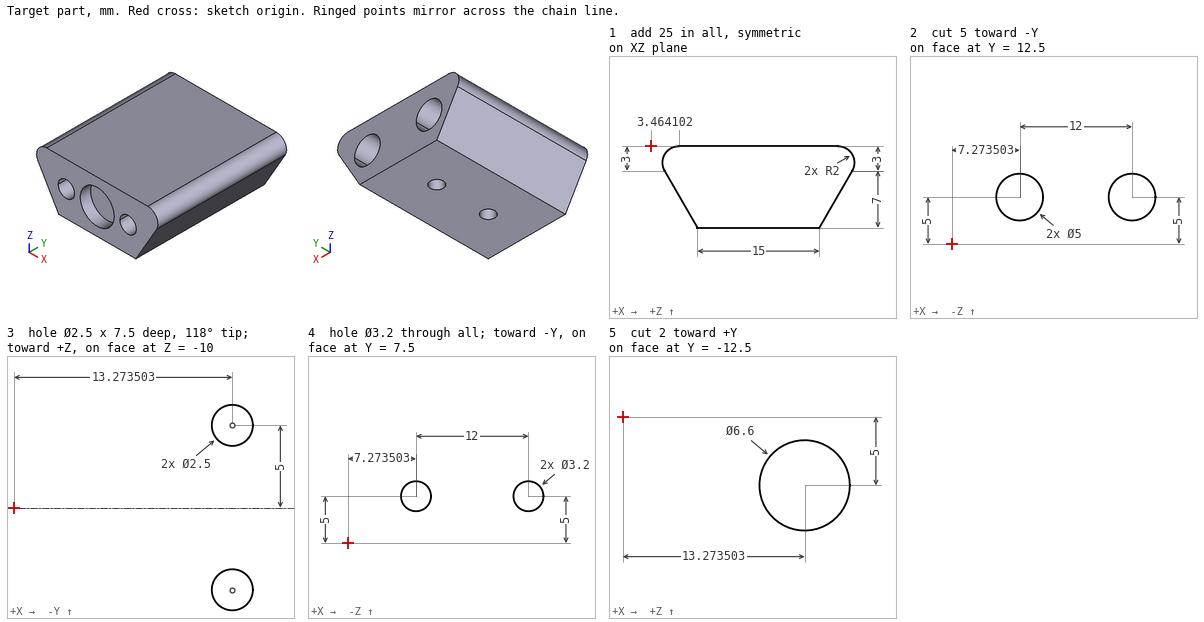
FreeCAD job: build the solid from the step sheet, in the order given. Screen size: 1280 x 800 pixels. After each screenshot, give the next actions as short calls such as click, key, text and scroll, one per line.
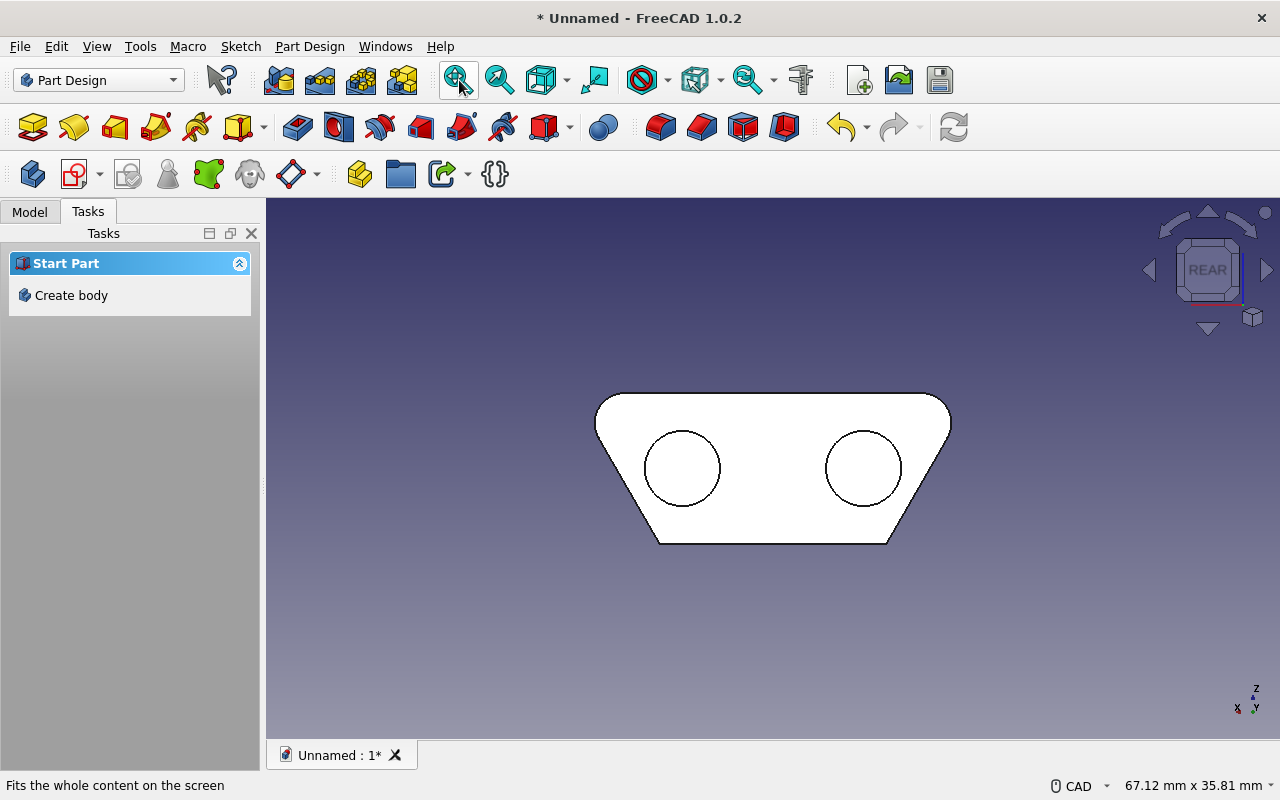
click(682, 467)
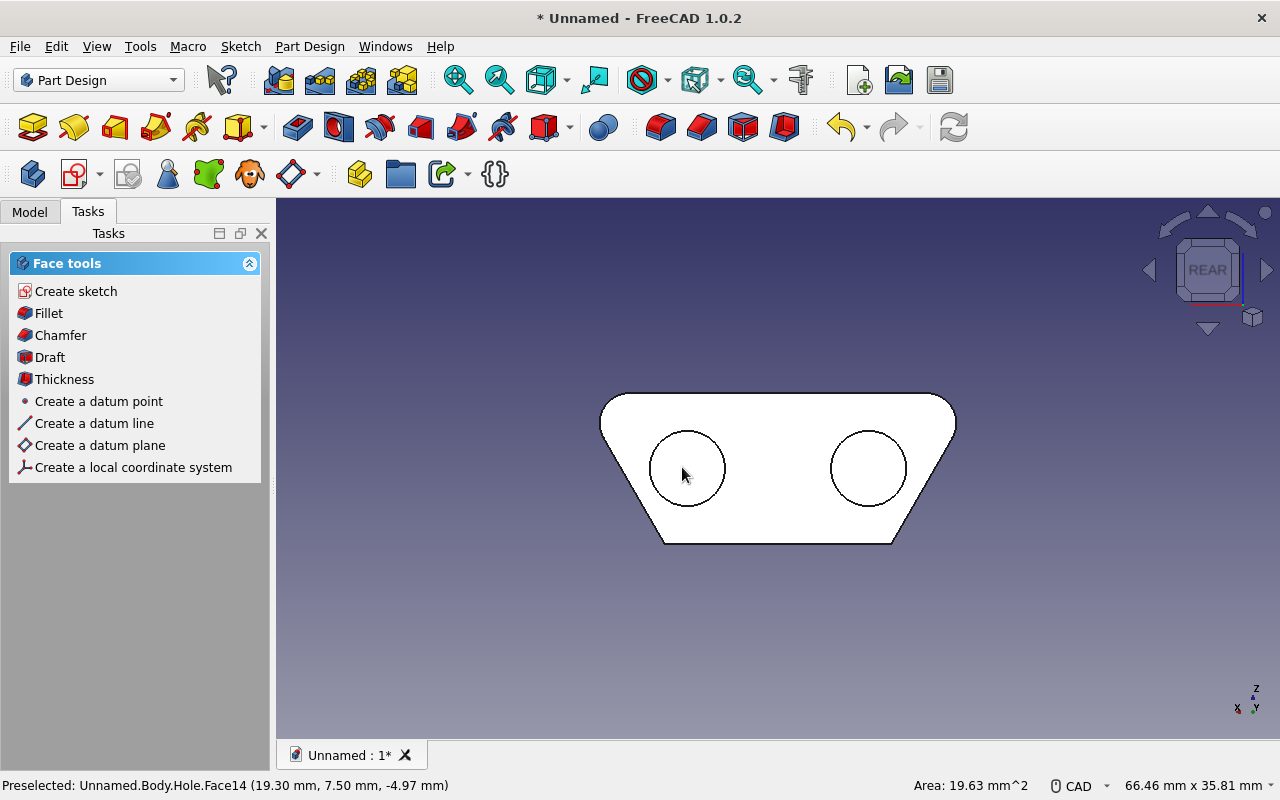
click(74, 174)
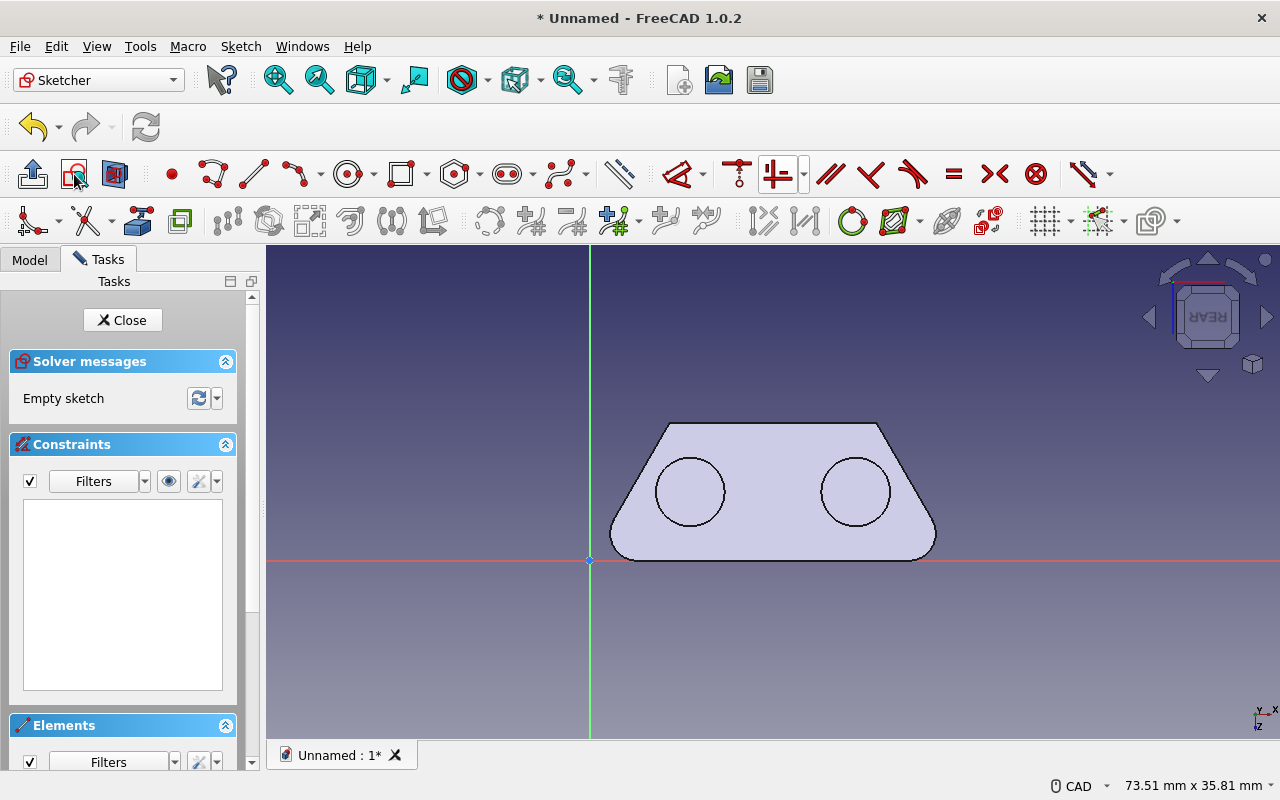
click(115, 174)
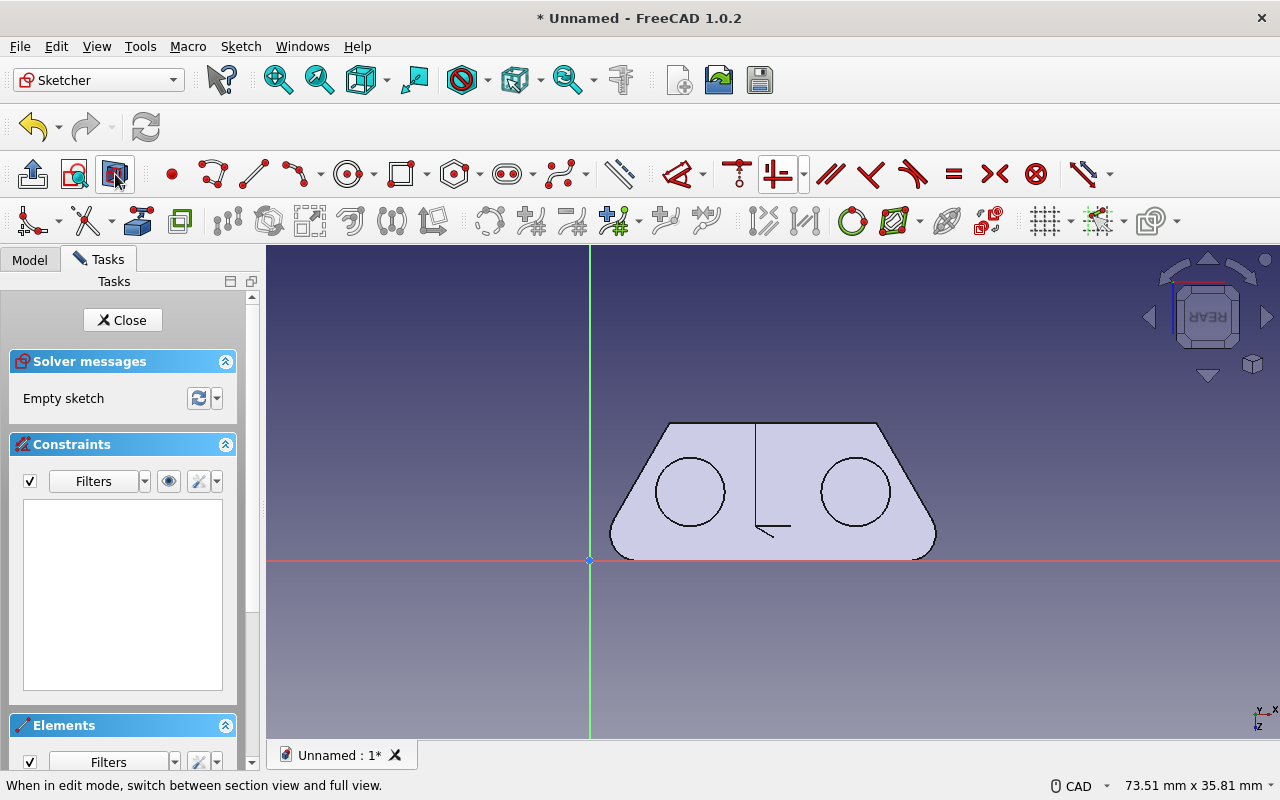
scroll(770, 544, up, 3)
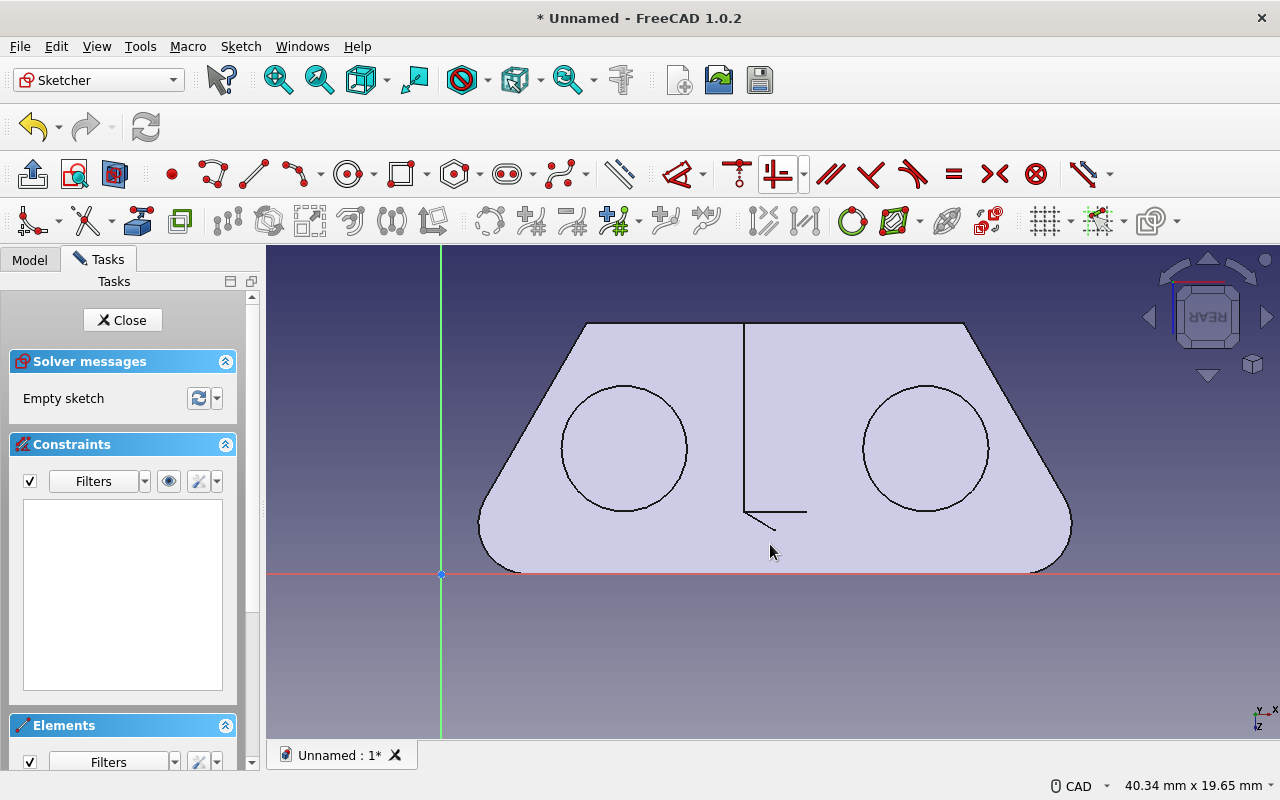
key(g)
key(c)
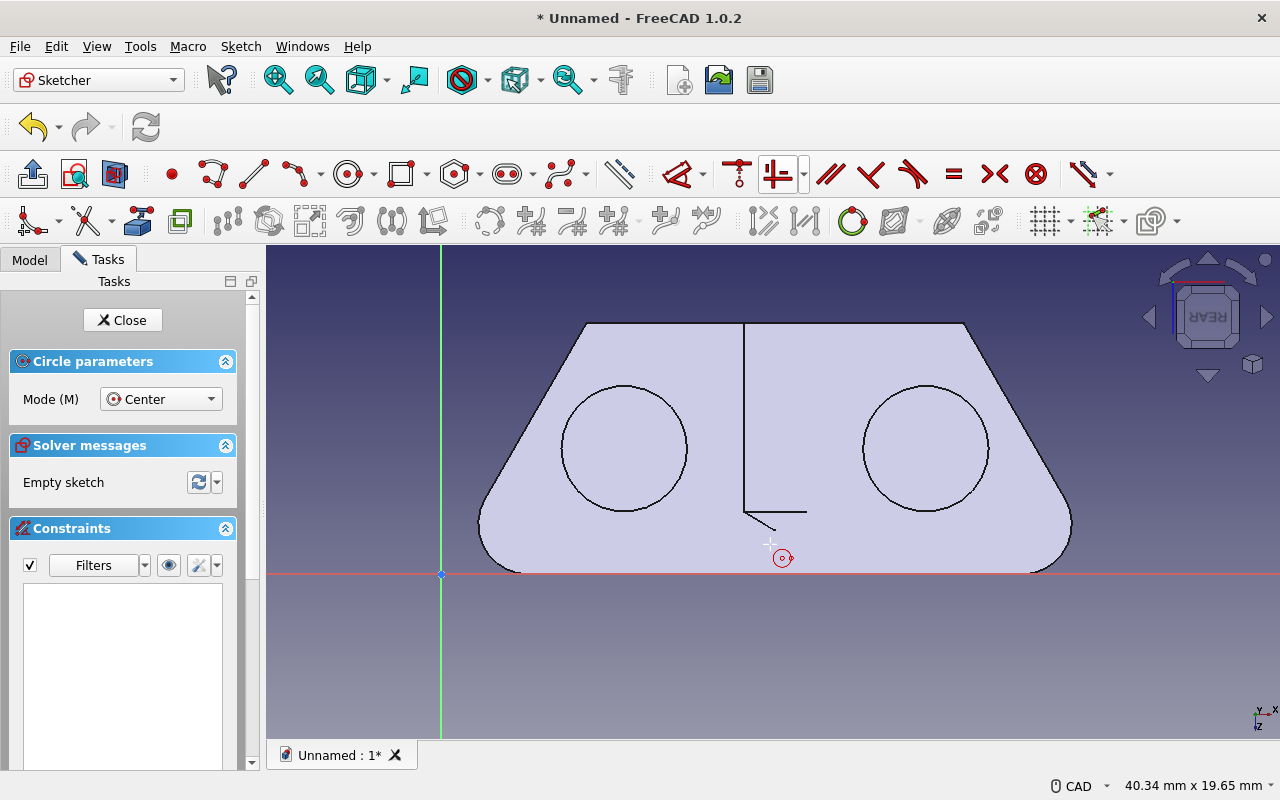
click(926, 449)
click(954, 420)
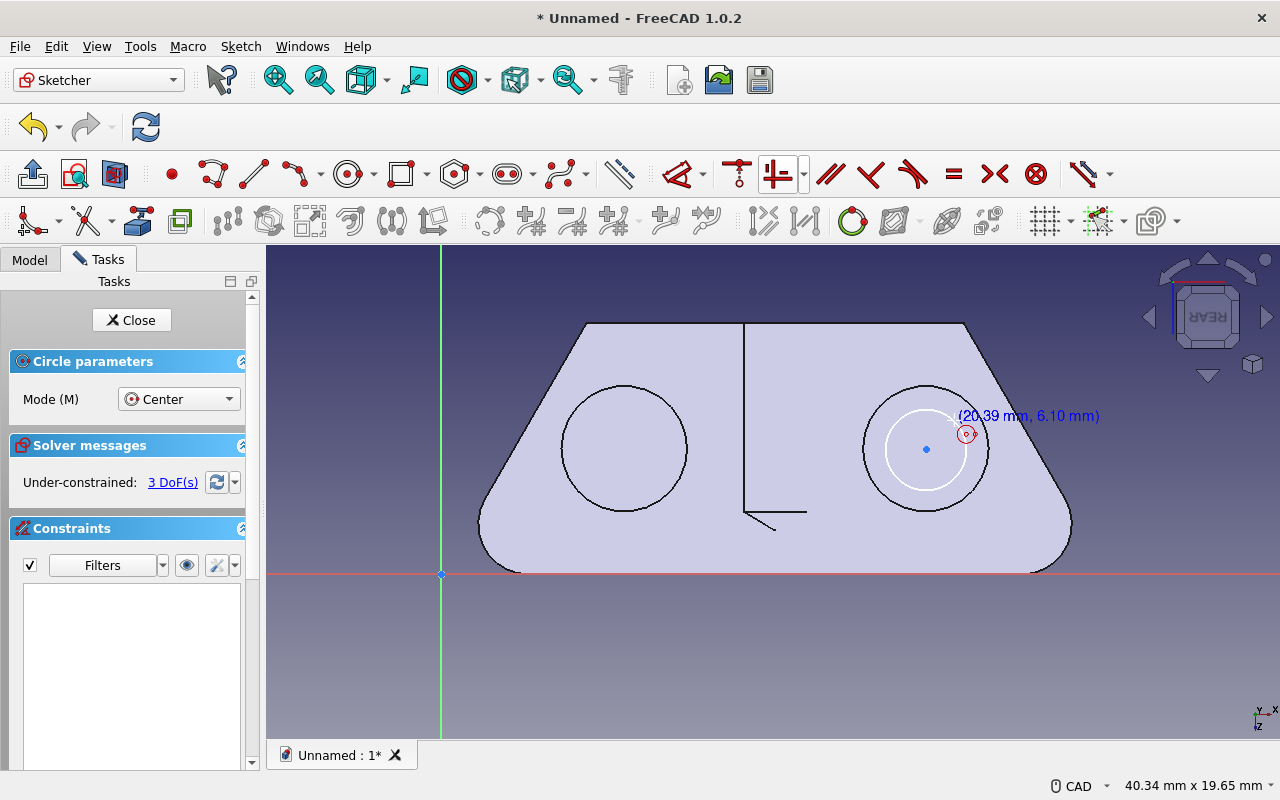
click(624, 449)
click(653, 420)
key(Escape)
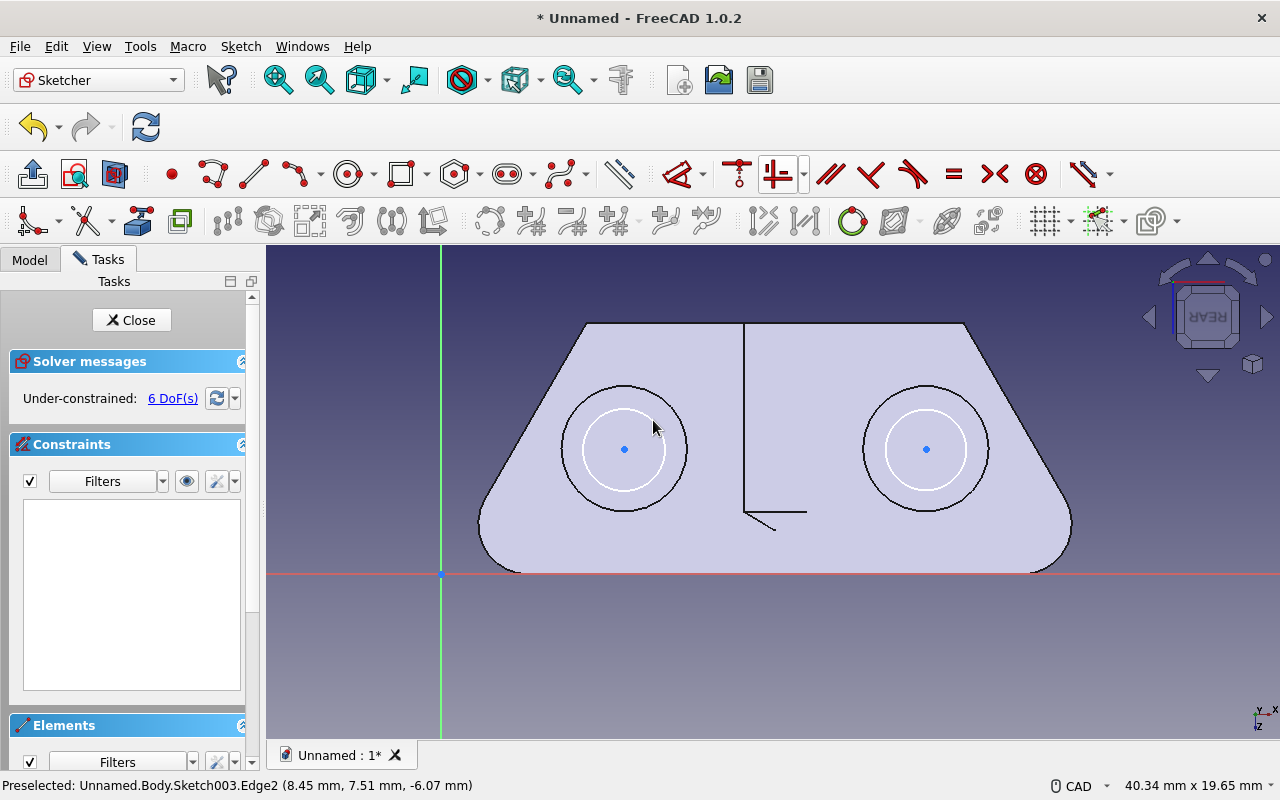
click(954, 421)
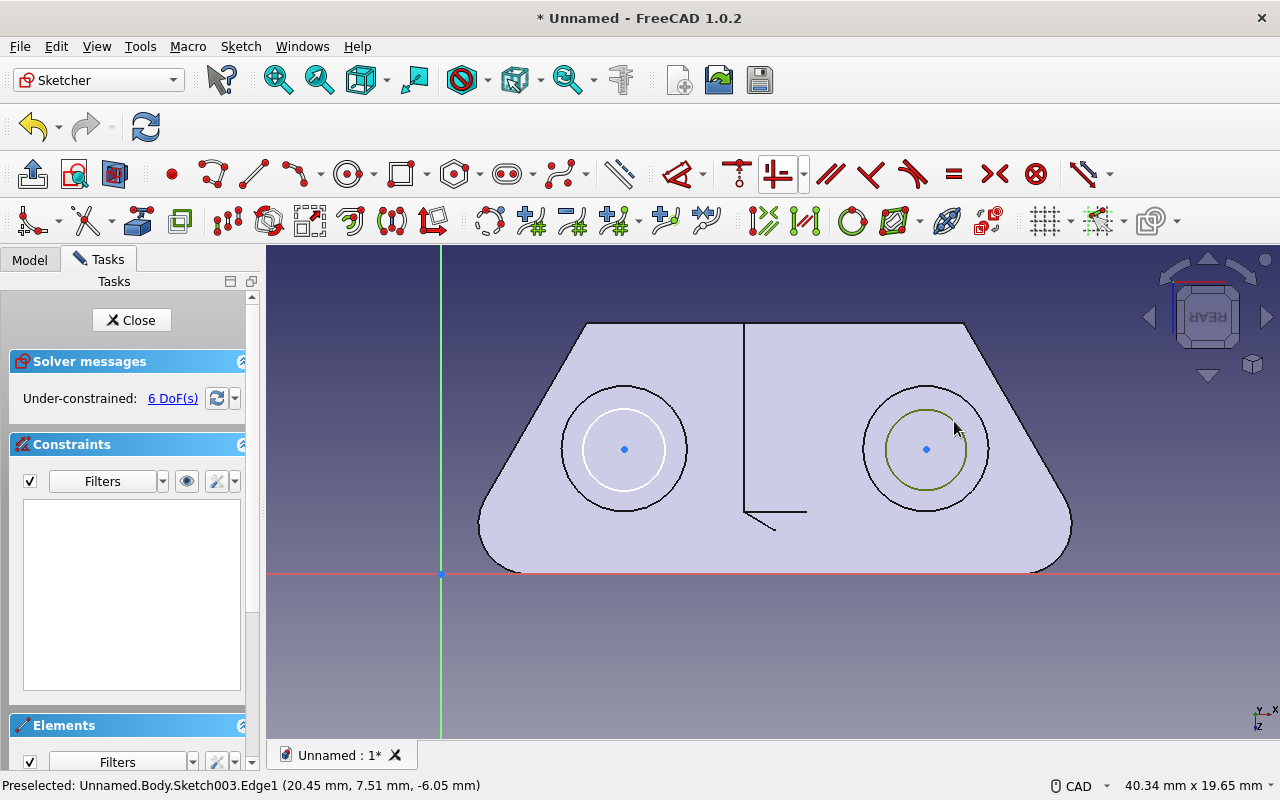
click(653, 421)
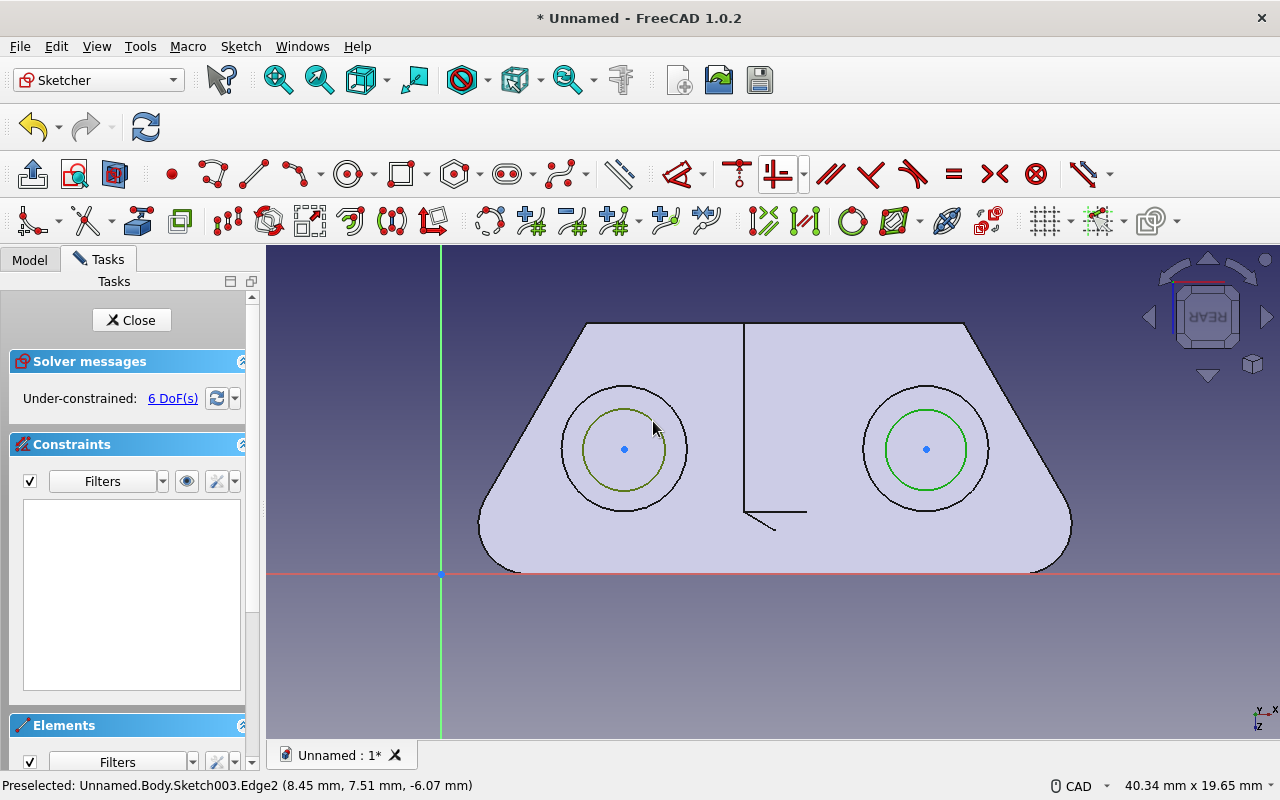
key(e)